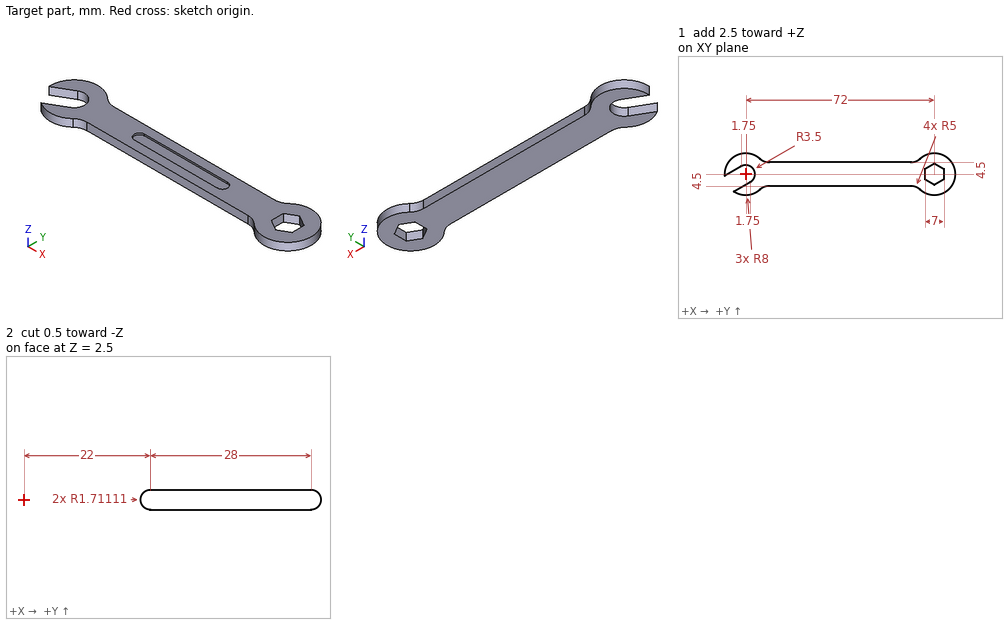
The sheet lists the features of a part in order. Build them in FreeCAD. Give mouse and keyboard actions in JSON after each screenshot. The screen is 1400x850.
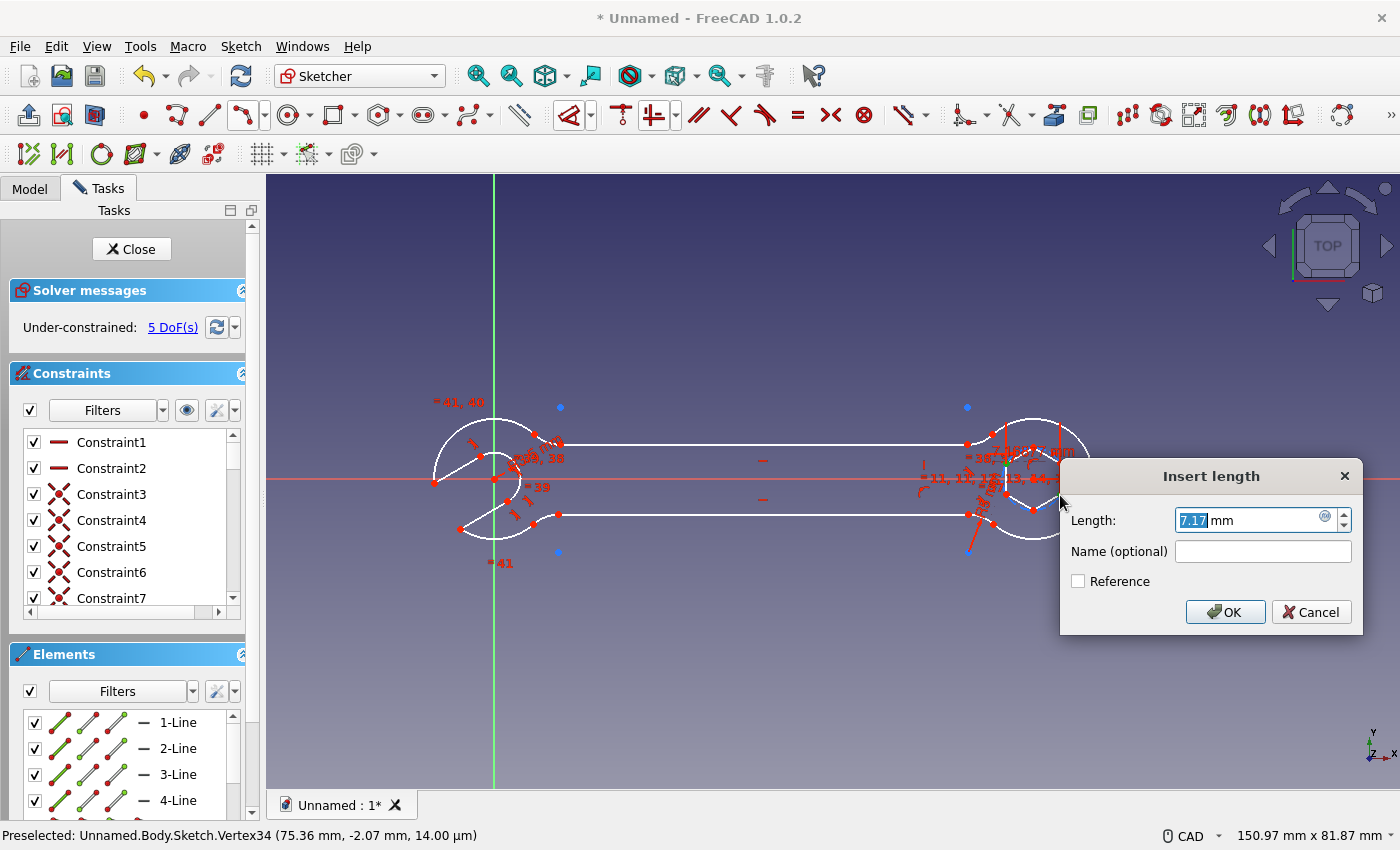
{"action": "type", "text": "7"}
{"action": "key", "text": "Return"}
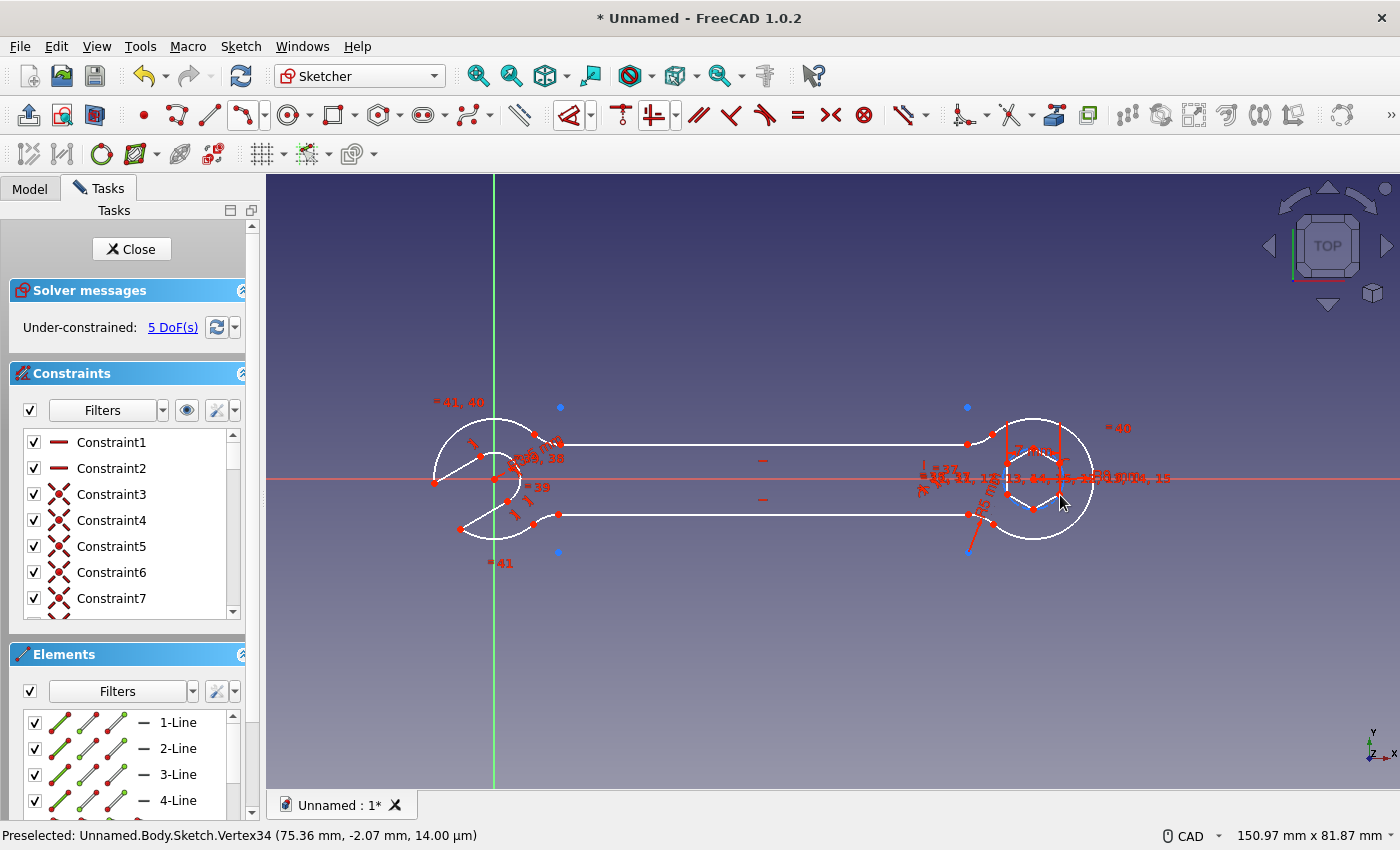
{"action": "left_click", "coordinate": [1033, 479]}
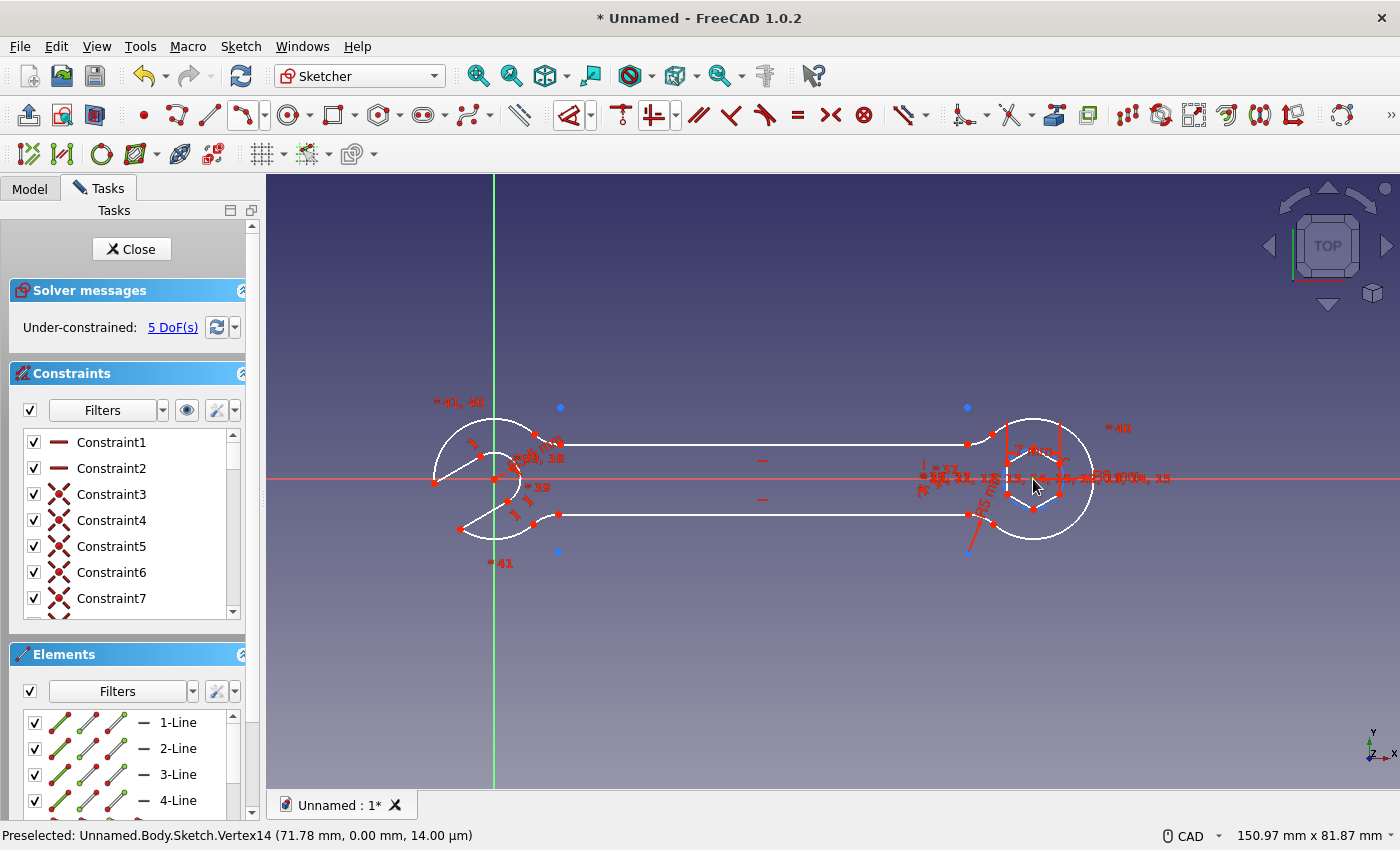
{"action": "left_click", "coordinate": [590, 116]}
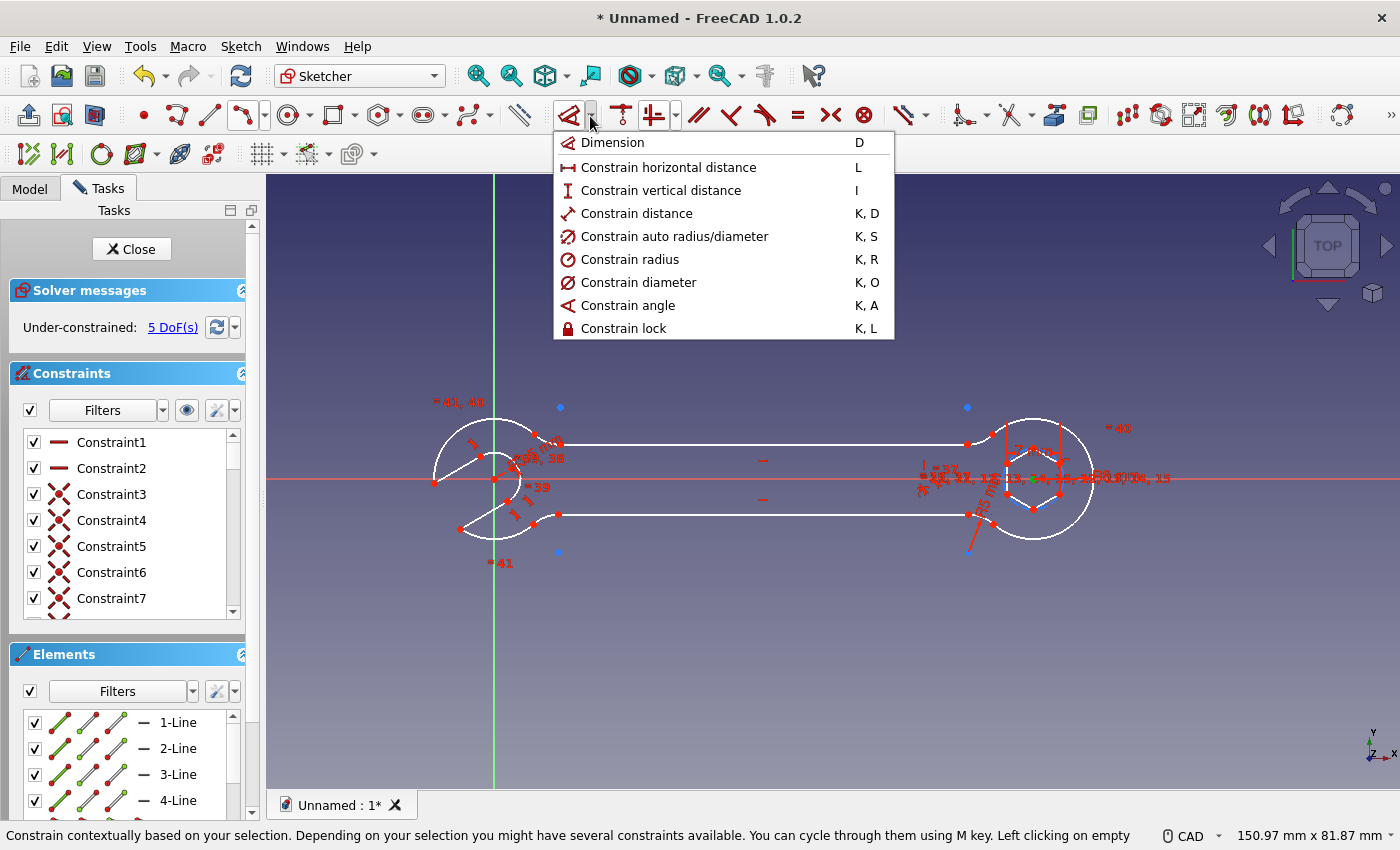
{"action": "left_click", "coordinate": [724, 168]}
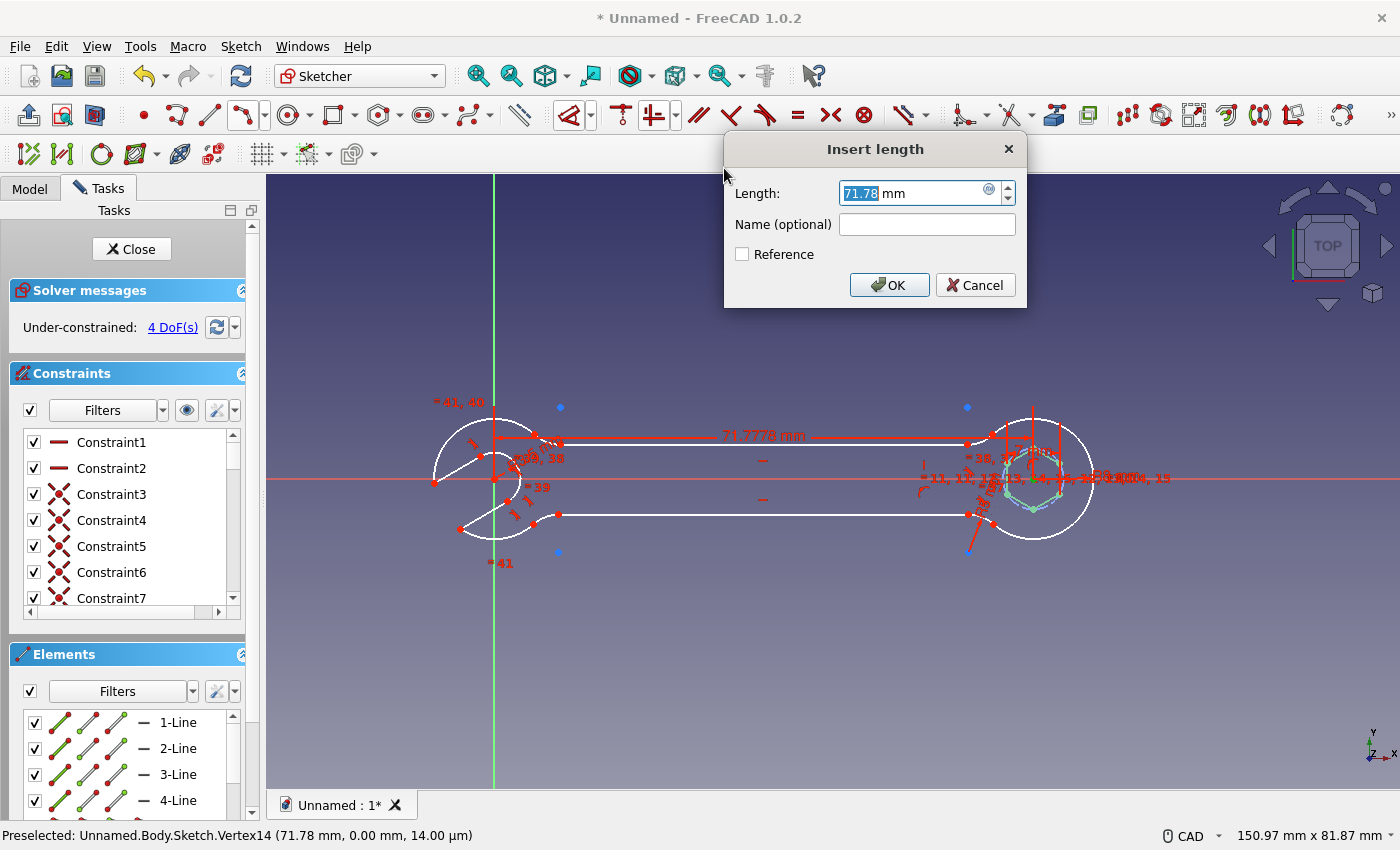
{"action": "type", "text": "72"}
{"action": "key", "text": "Return"}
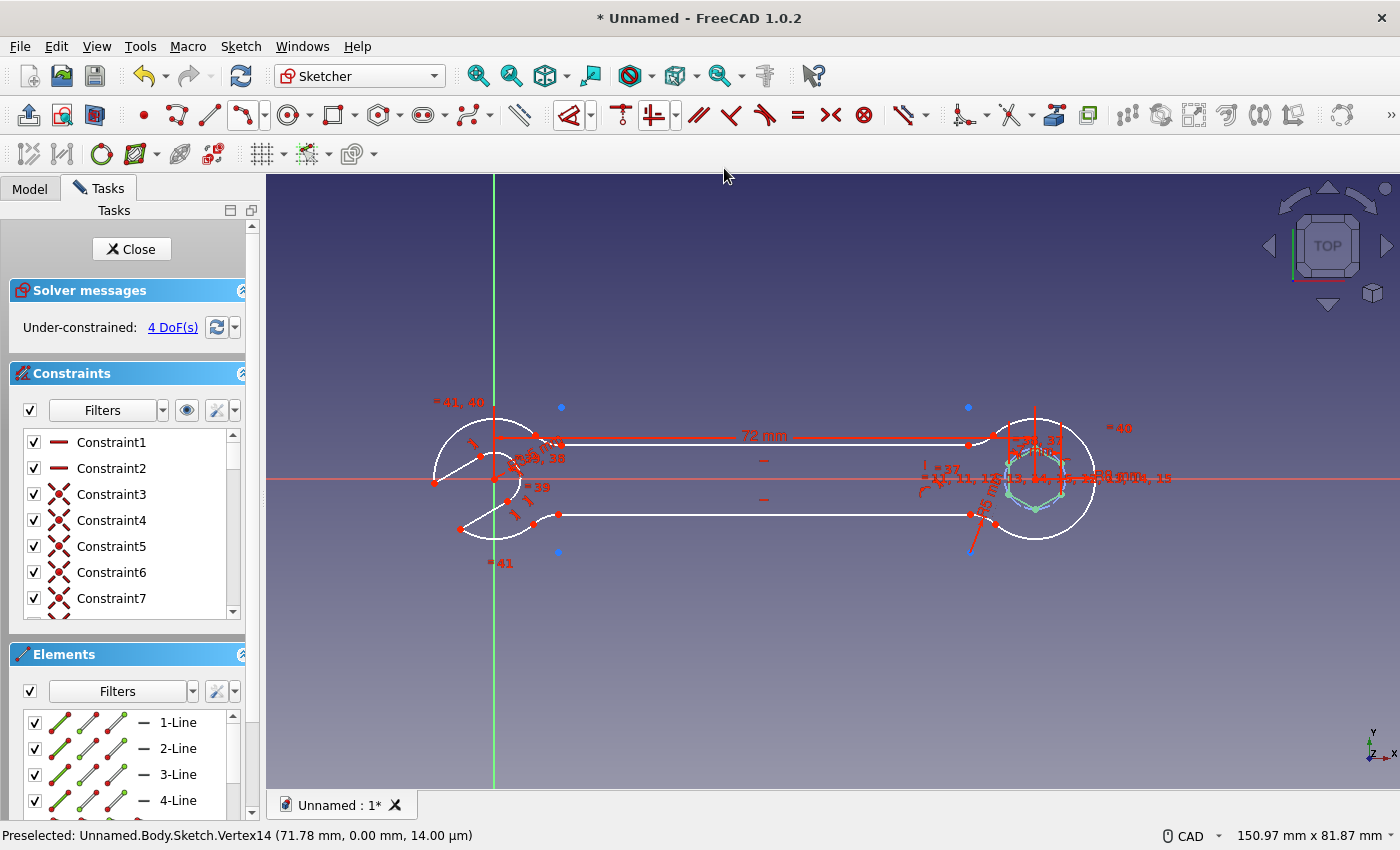
{"action": "left_click", "coordinate": [559, 515]}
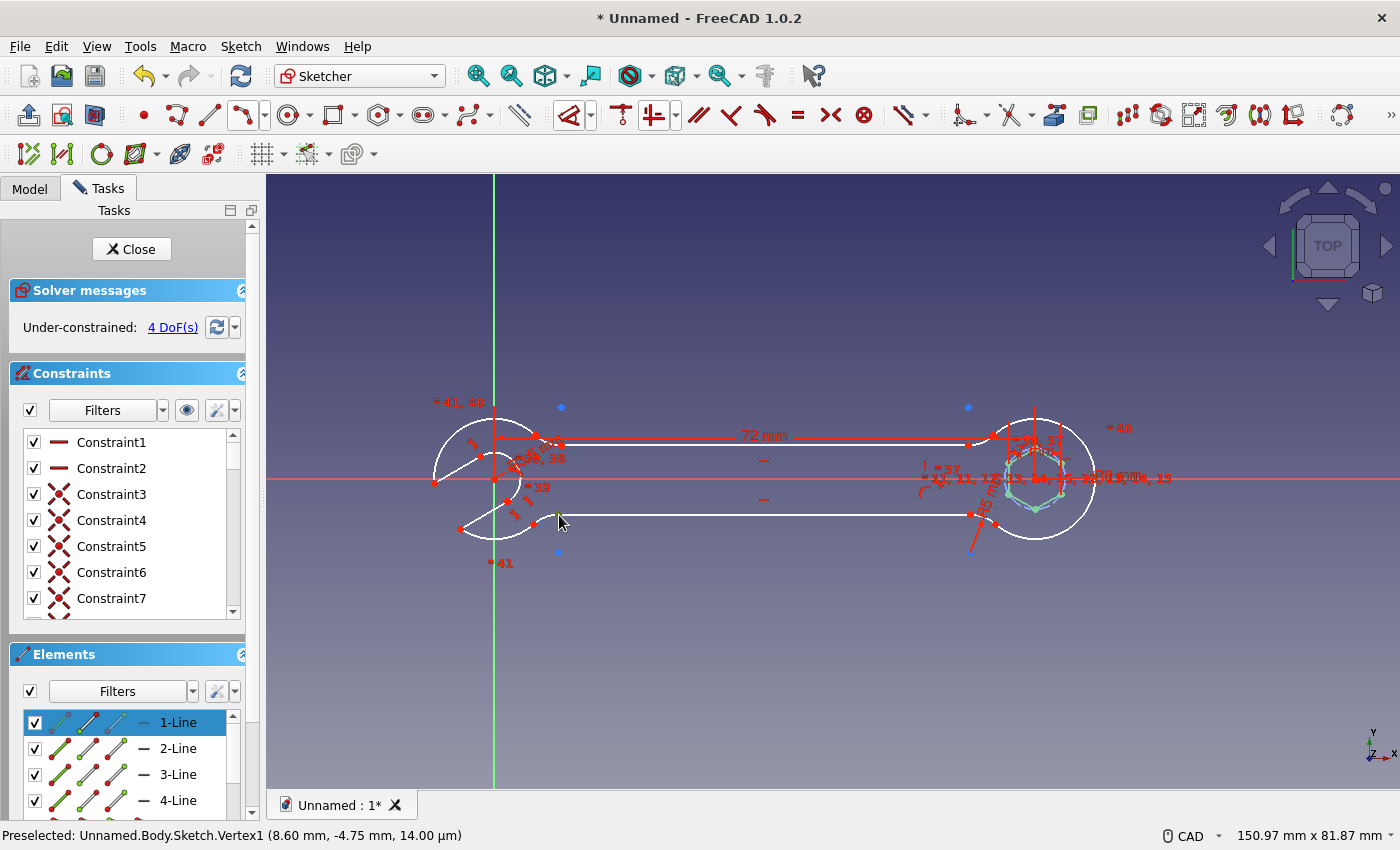
{"action": "key", "text": "i"}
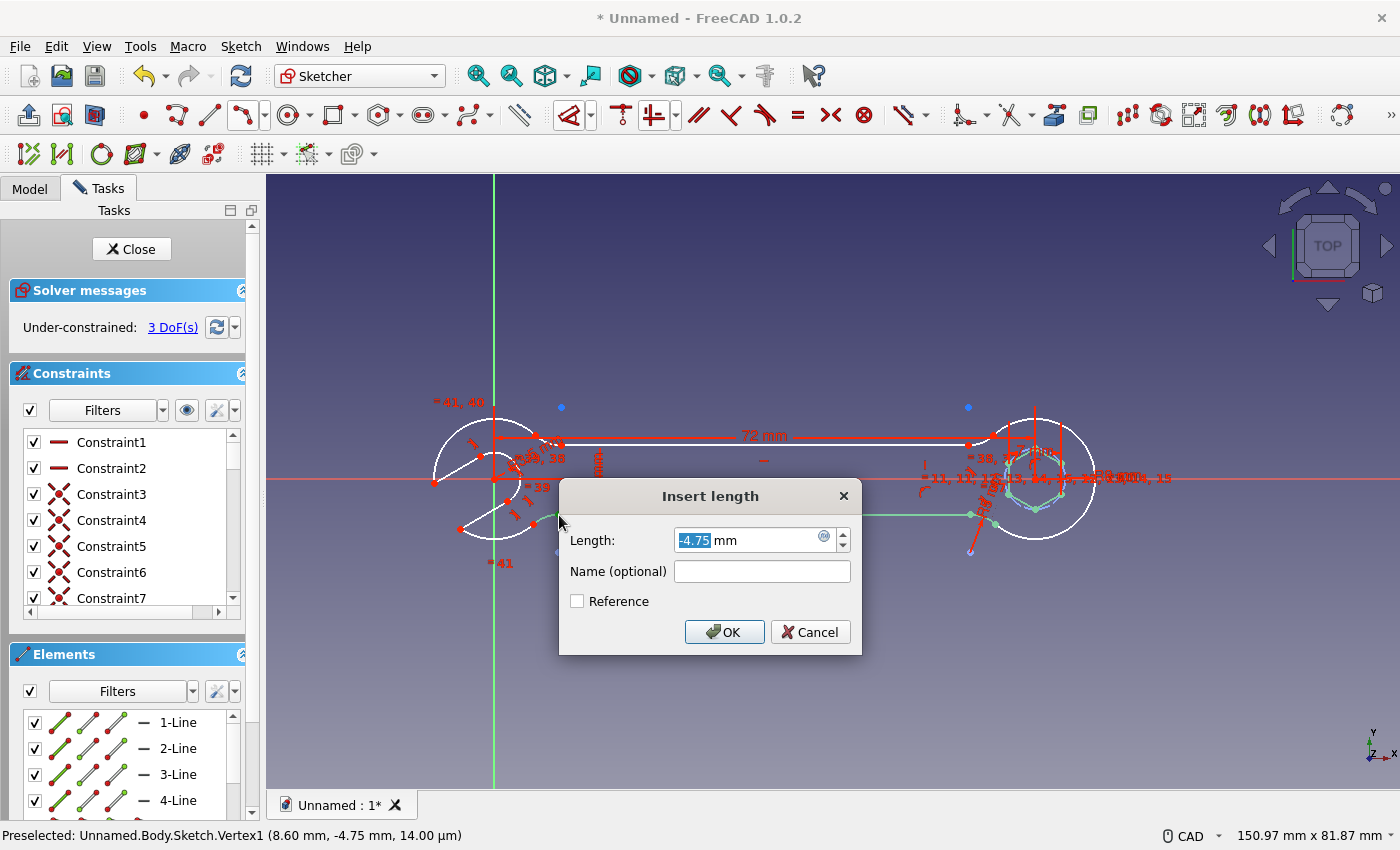
{"action": "type", "text": "-4.5"}
{"action": "key", "text": "Return"}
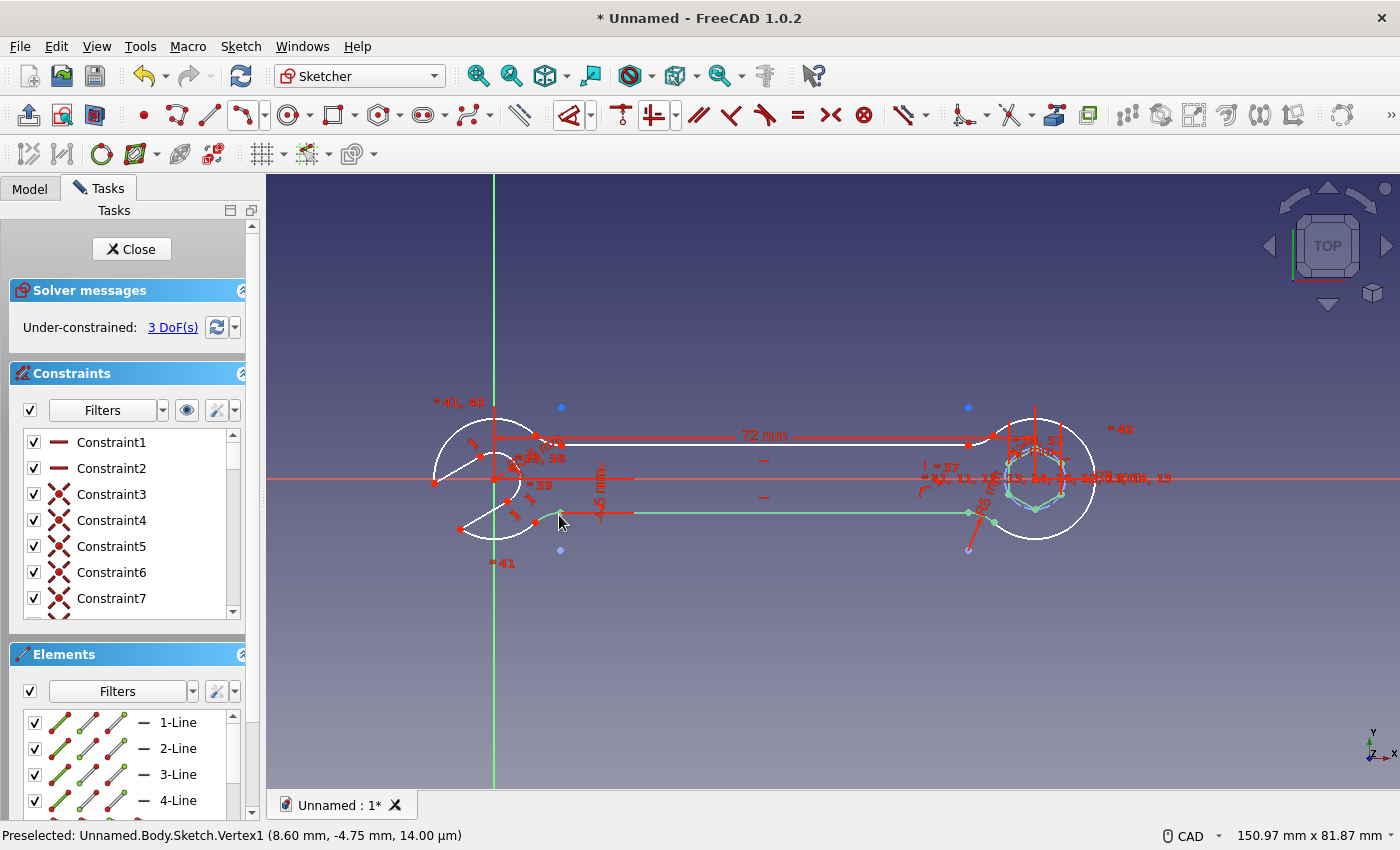
{"action": "left_click", "coordinate": [968, 445]}